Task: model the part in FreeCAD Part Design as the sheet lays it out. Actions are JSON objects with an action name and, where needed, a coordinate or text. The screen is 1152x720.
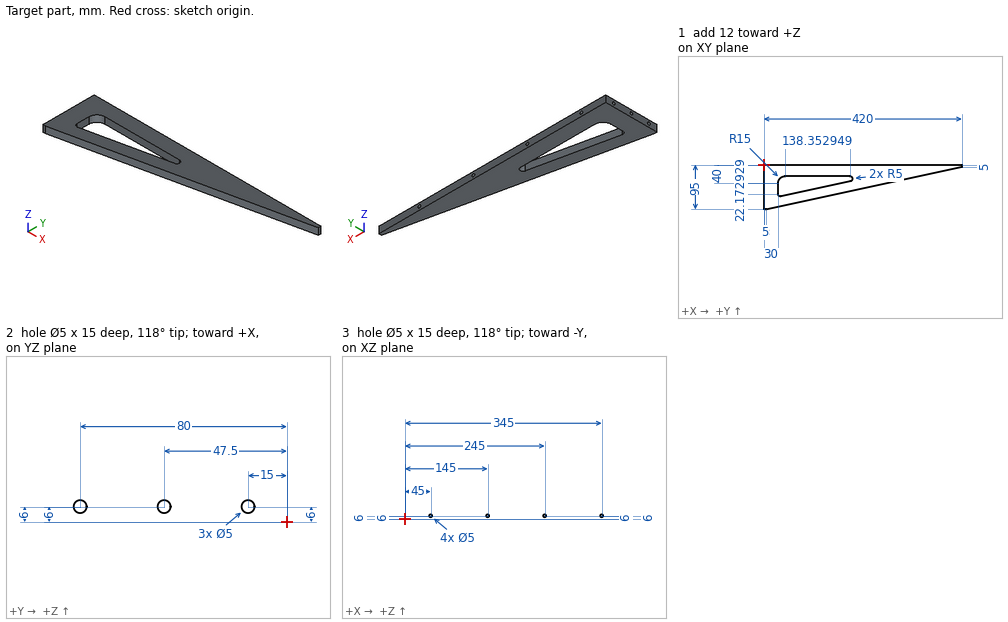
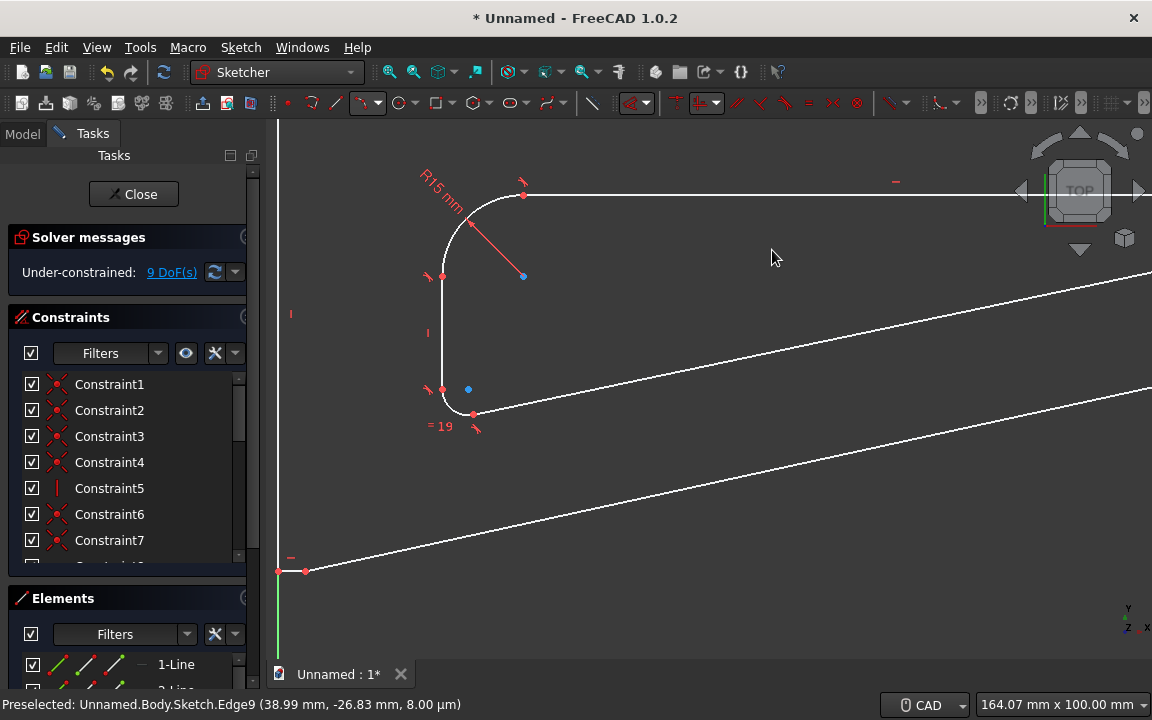
{"action": "scroll", "coordinate": [445, 409], "scroll_direction": "down", "scroll_amount": 8}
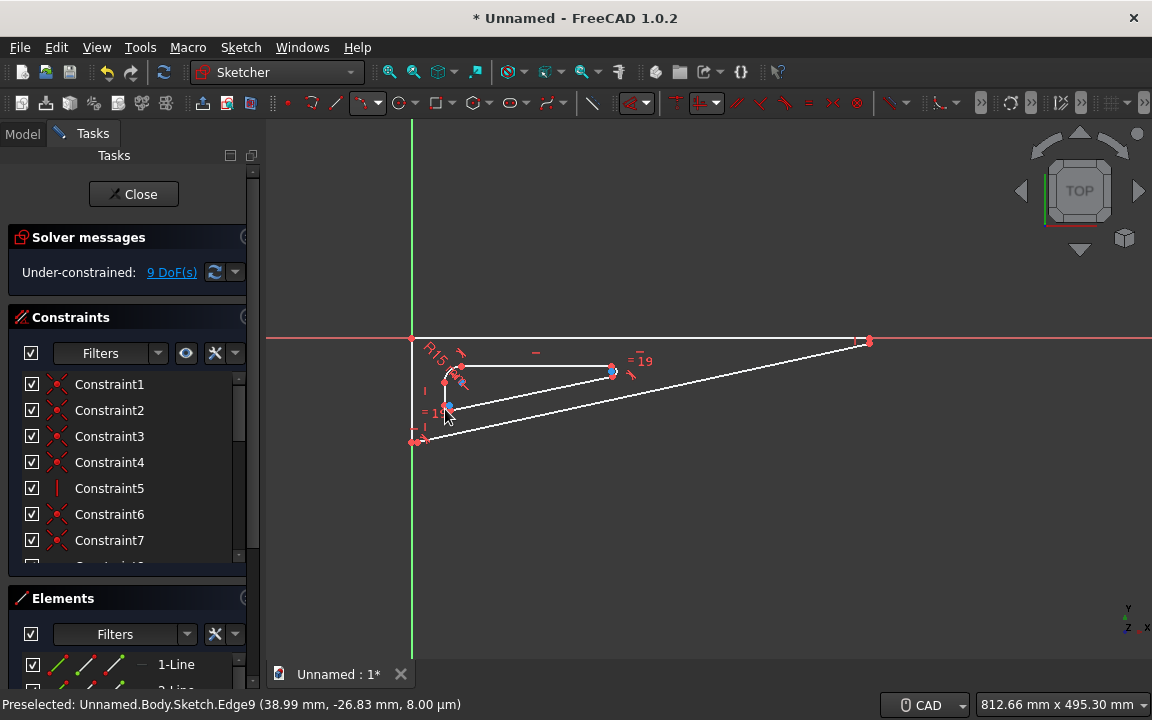
{"action": "scroll", "coordinate": [616, 374], "scroll_direction": "up", "scroll_amount": 10}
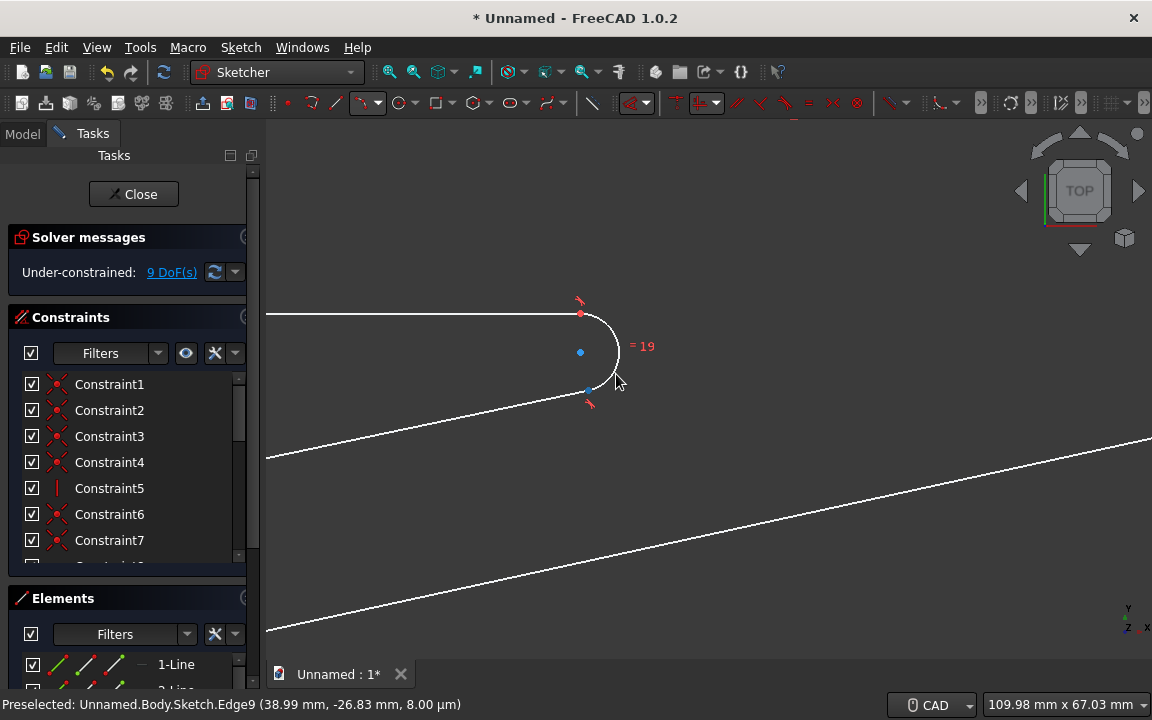
{"action": "left_click", "coordinate": [615, 371]}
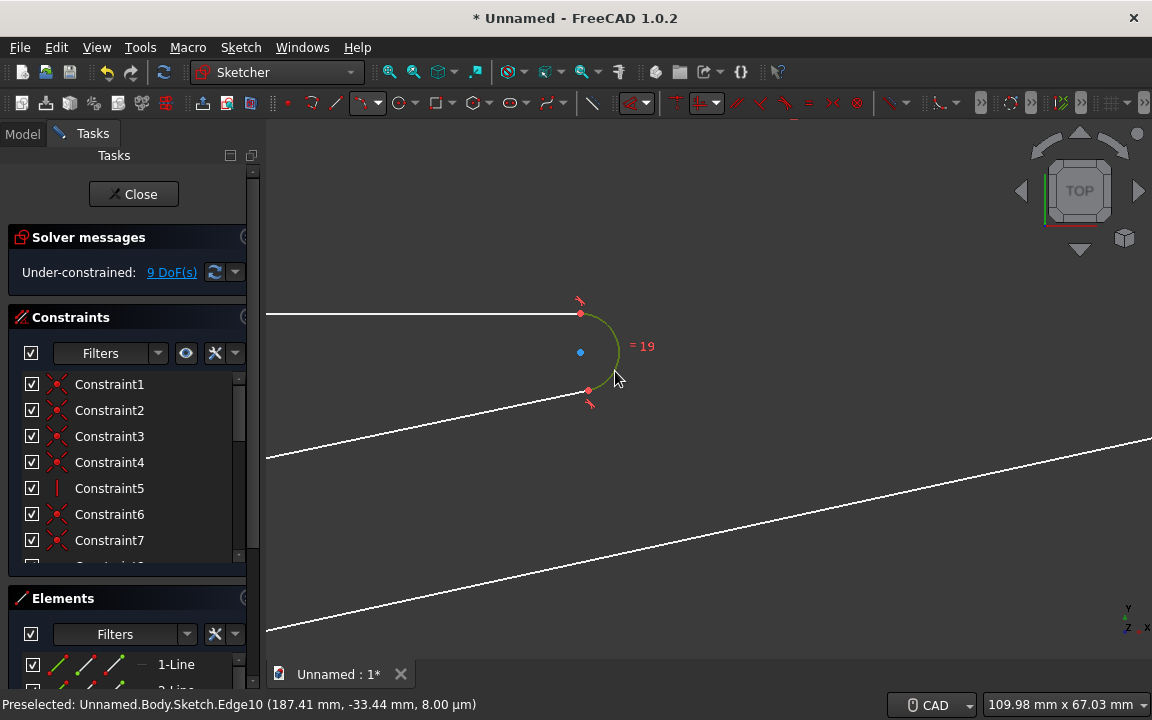
{"action": "key", "text": "k r"}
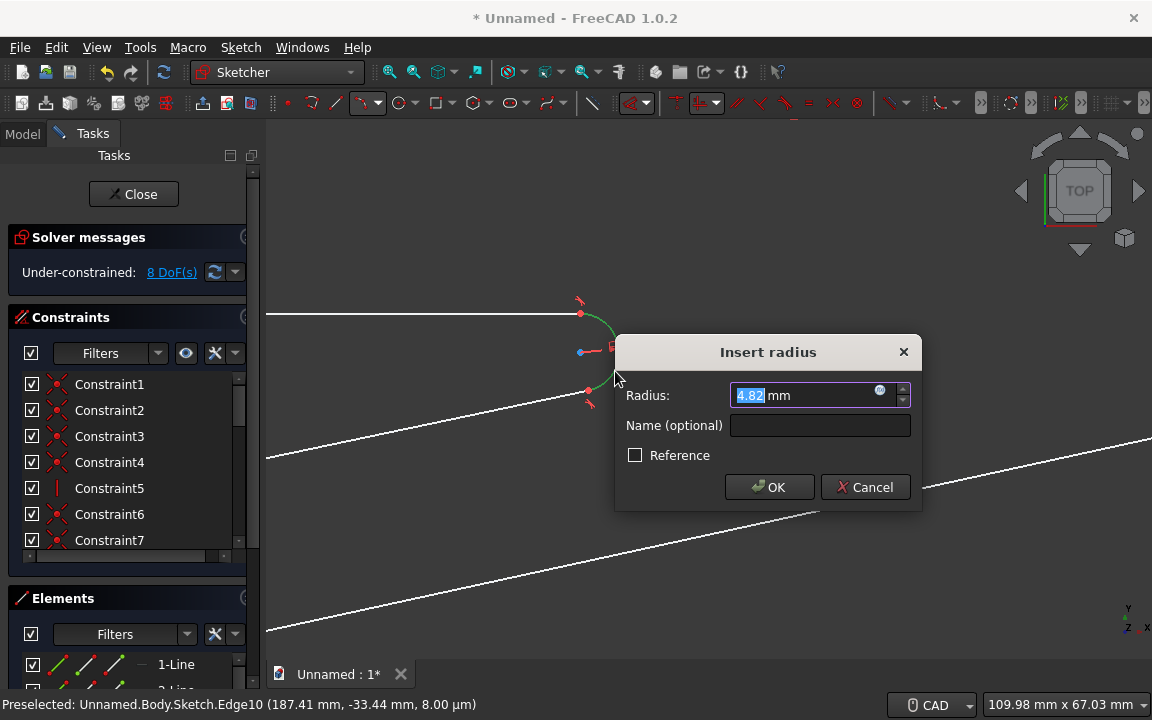
{"action": "type", "text": "5"}
{"action": "key", "text": "Return"}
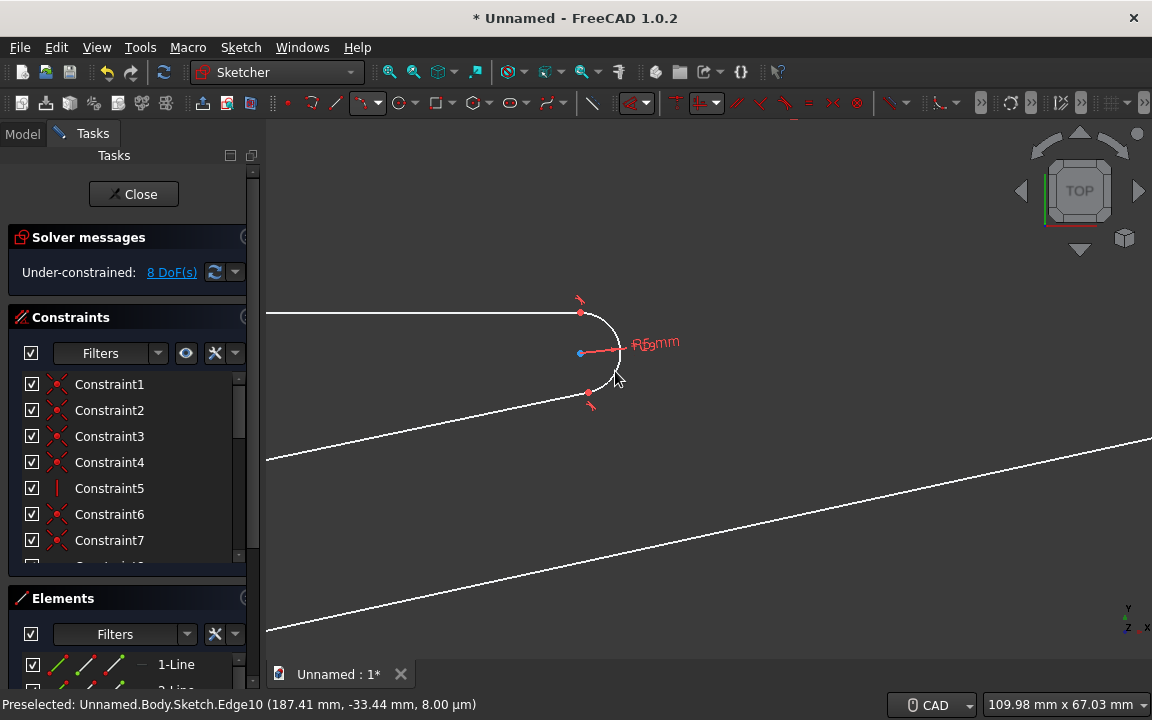
{"action": "scroll", "coordinate": [616, 374], "scroll_direction": "down", "scroll_amount": 10}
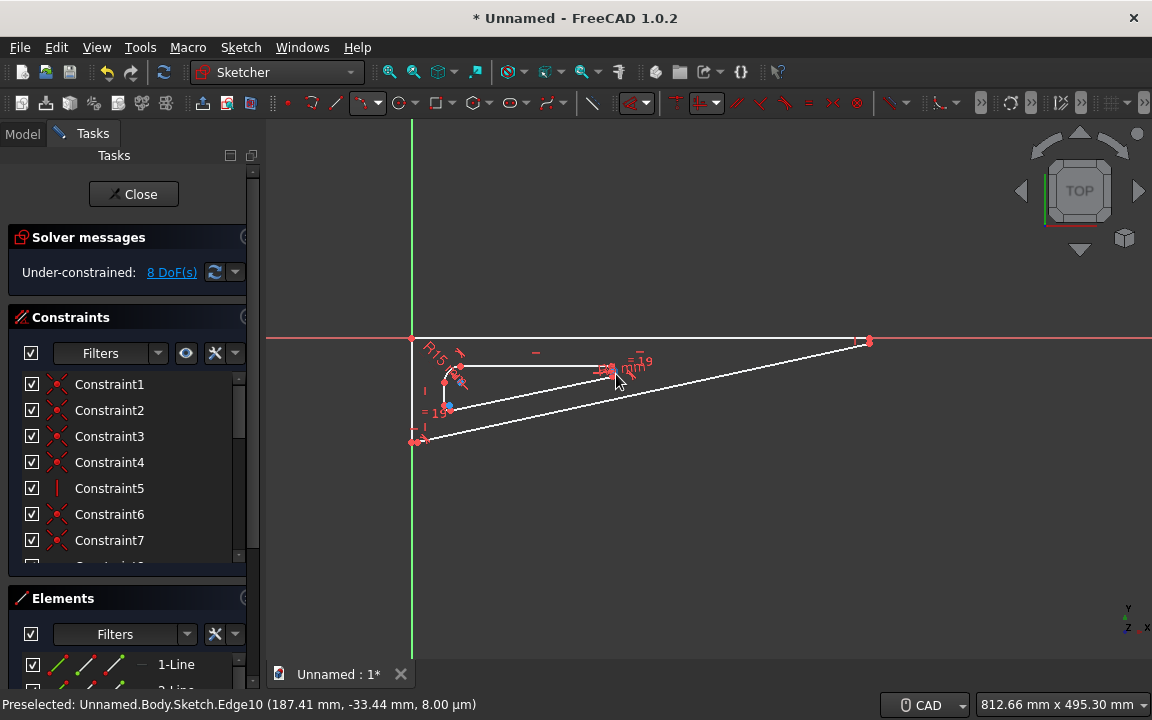
{"action": "scroll", "coordinate": [413, 442], "scroll_direction": "up", "scroll_amount": 11}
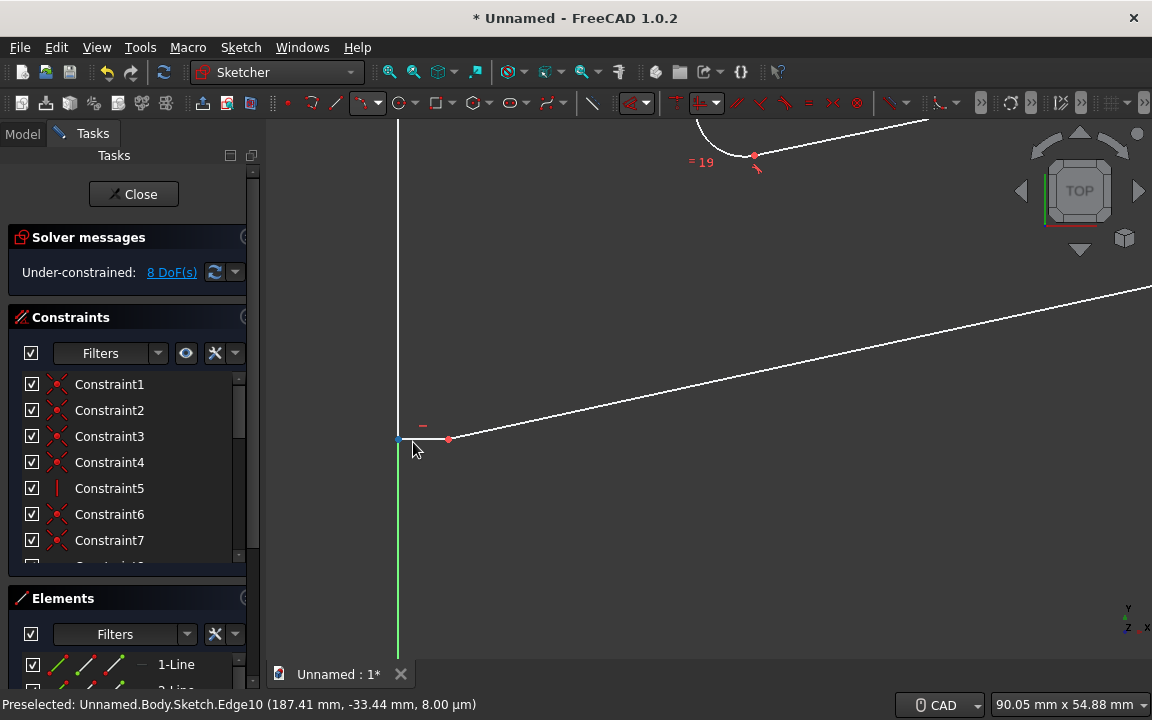
{"action": "left_click", "coordinate": [413, 439]}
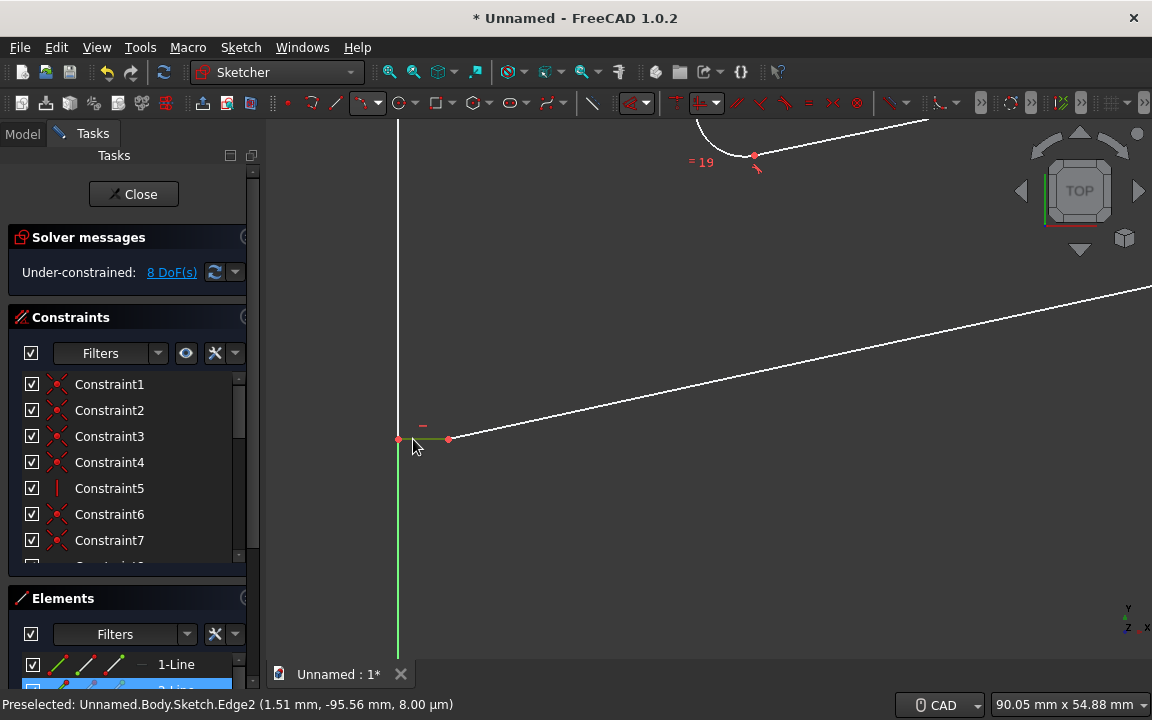
{"action": "key", "text": "l"}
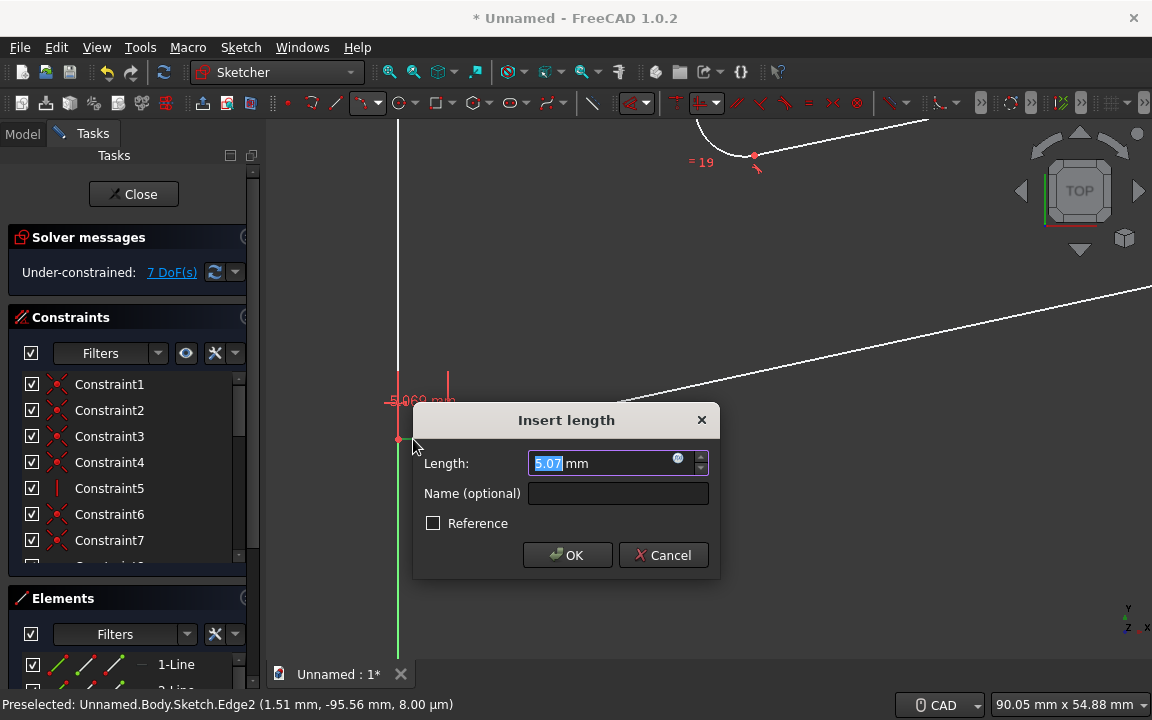
{"action": "type", "text": "5"}
{"action": "key", "text": "Return"}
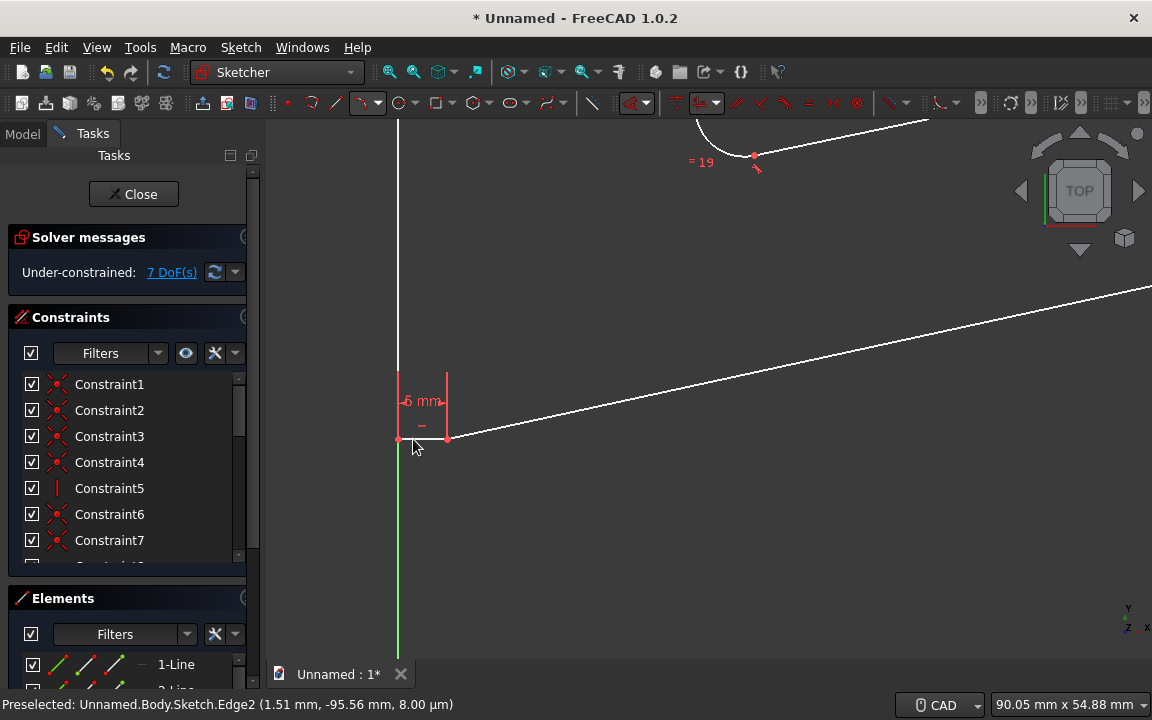
{"action": "scroll", "coordinate": [413, 442], "scroll_direction": "down", "scroll_amount": 11}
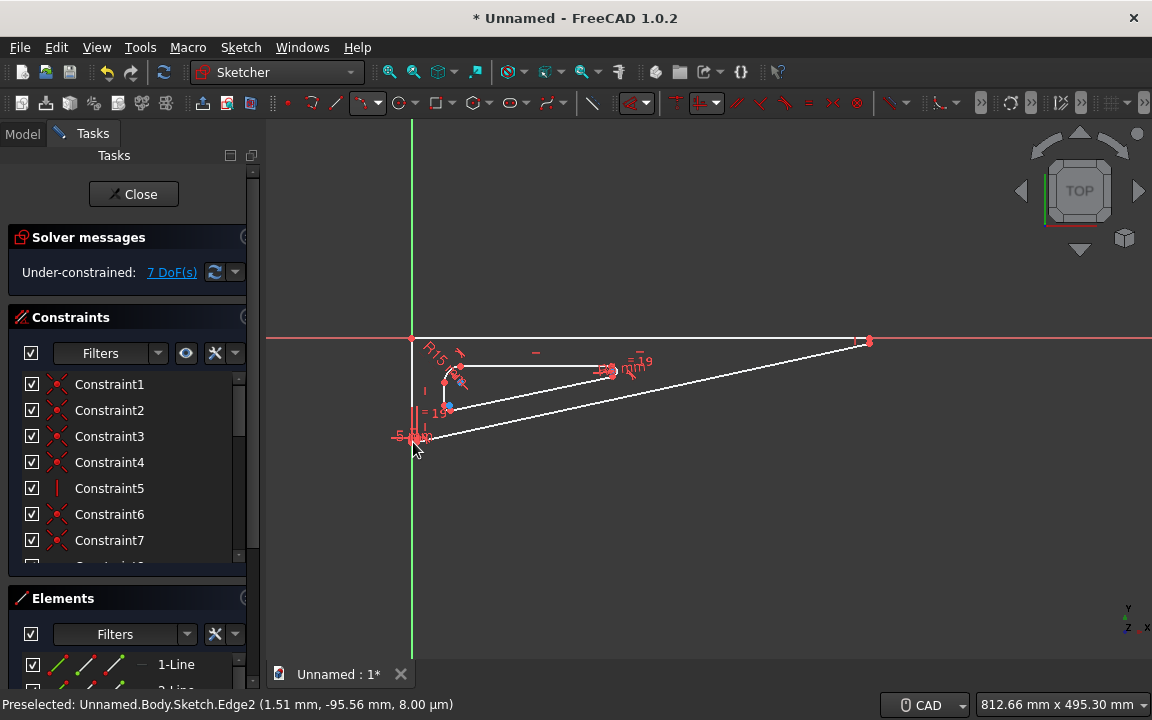
{"action": "scroll", "coordinate": [869, 342], "scroll_direction": "up", "scroll_amount": 11}